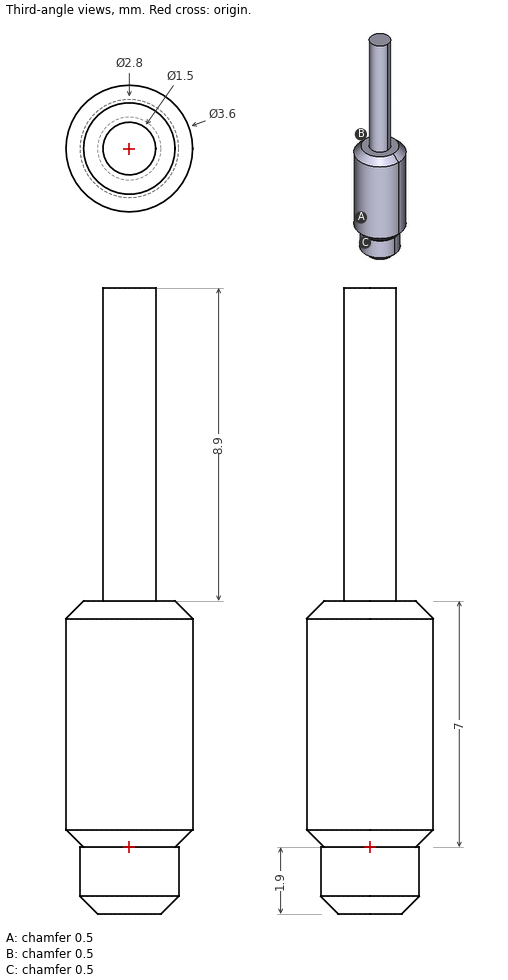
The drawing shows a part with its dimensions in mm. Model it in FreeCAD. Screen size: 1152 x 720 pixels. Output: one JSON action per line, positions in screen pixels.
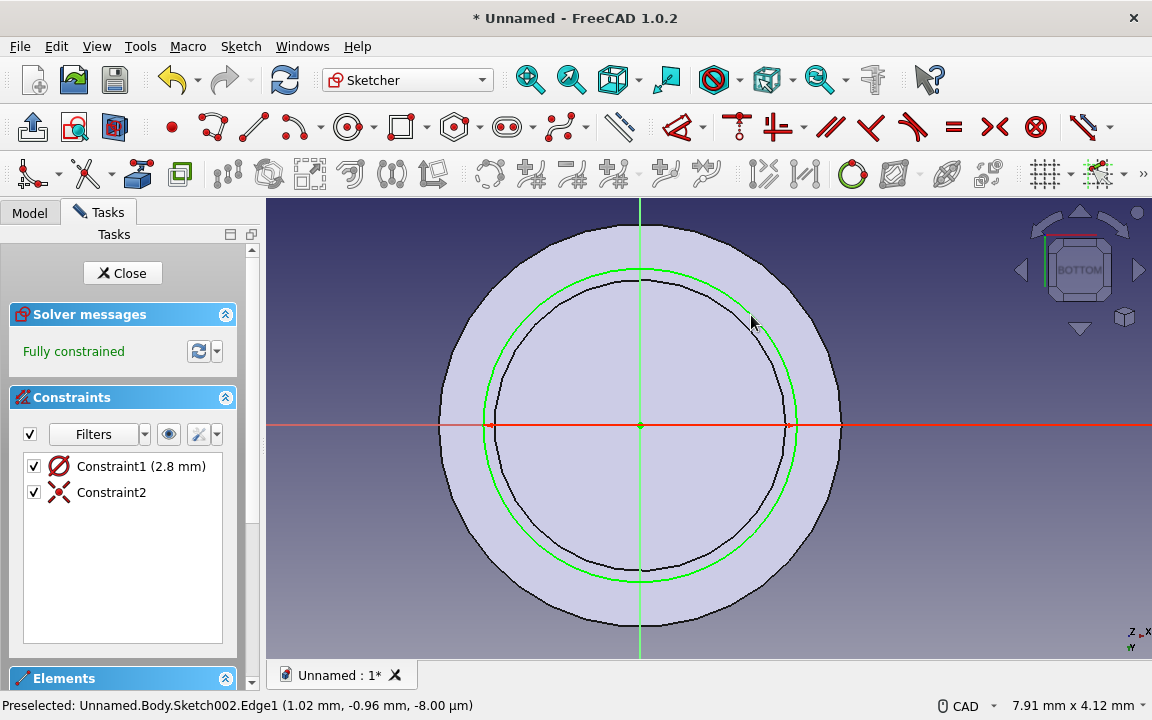
{"action": "left_click", "coordinate": [123, 273]}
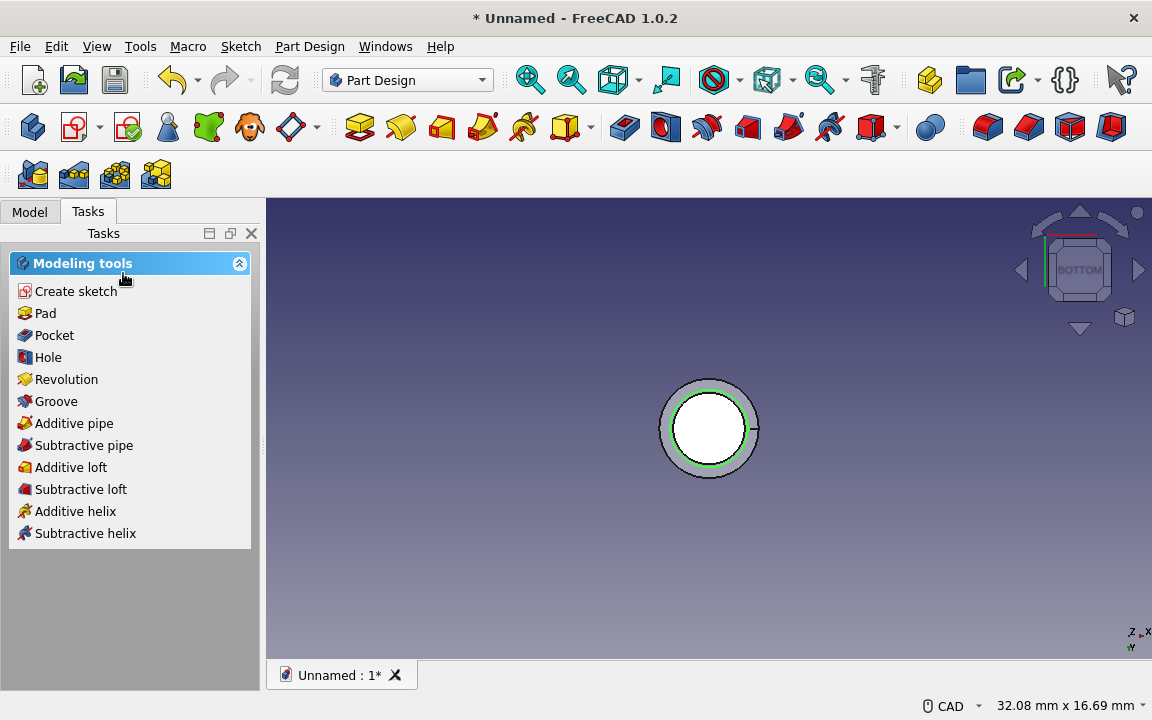
{"action": "left_click", "coordinate": [360, 128]}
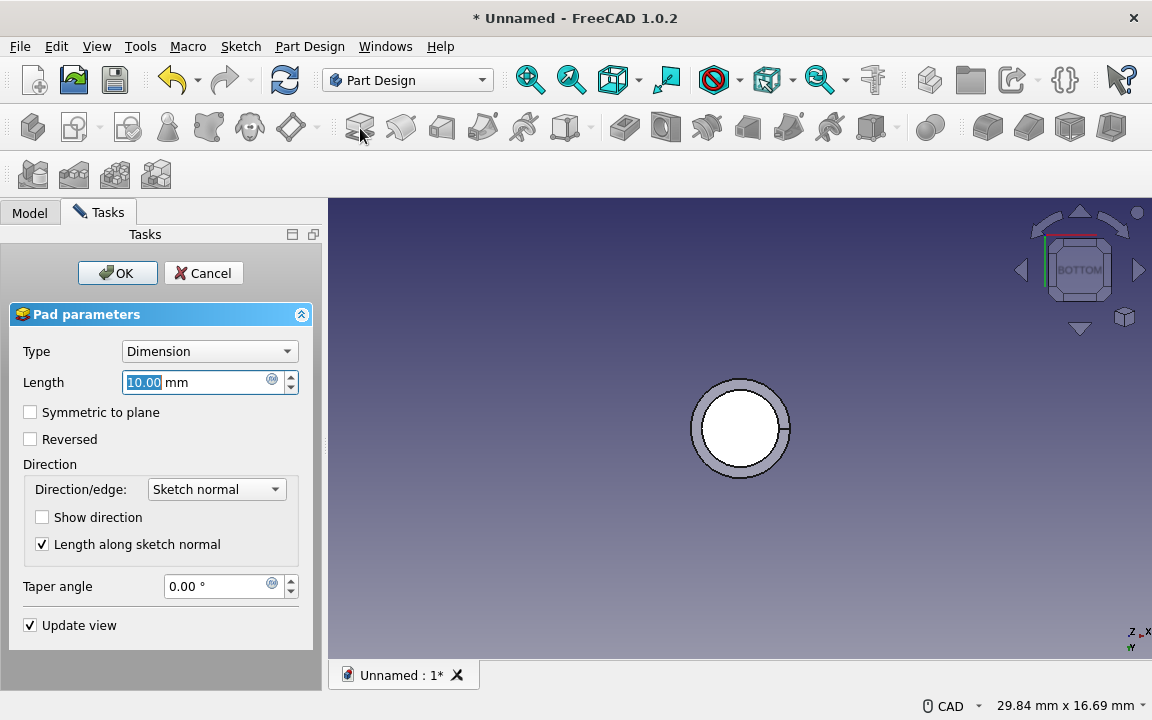
{"action": "type", "text": "1.9"}
{"action": "key", "text": "Tab"}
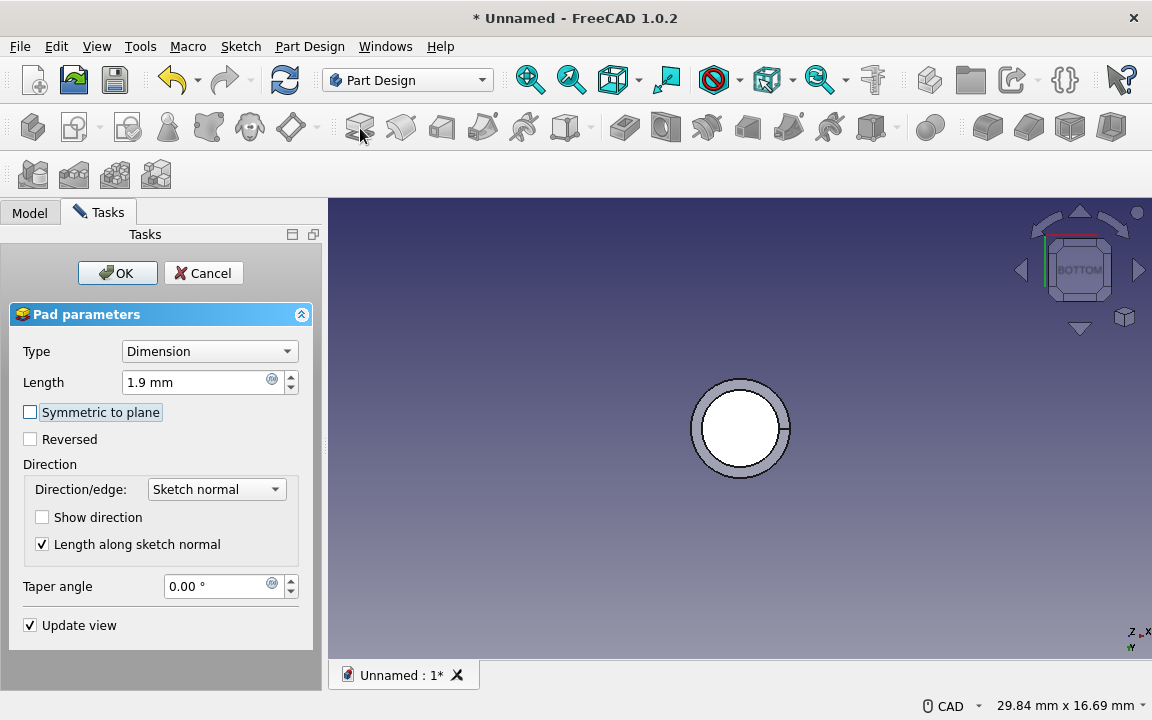
{"action": "left_click", "coordinate": [118, 273]}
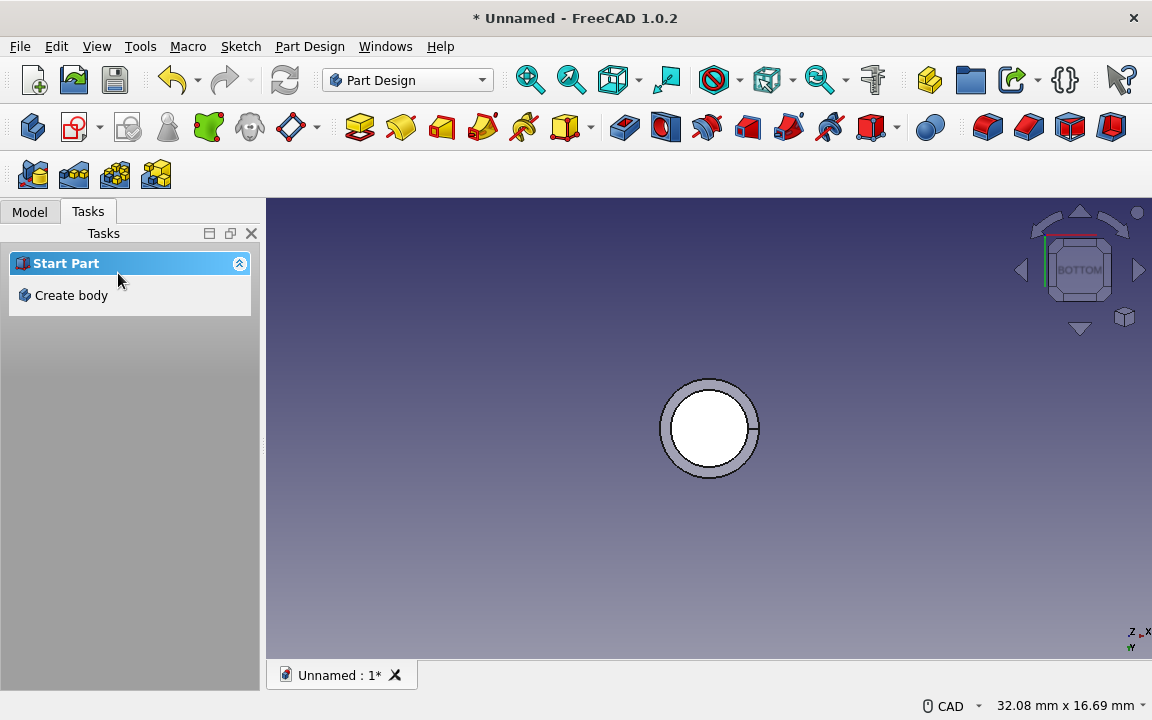
{"action": "key", "text": "v f"}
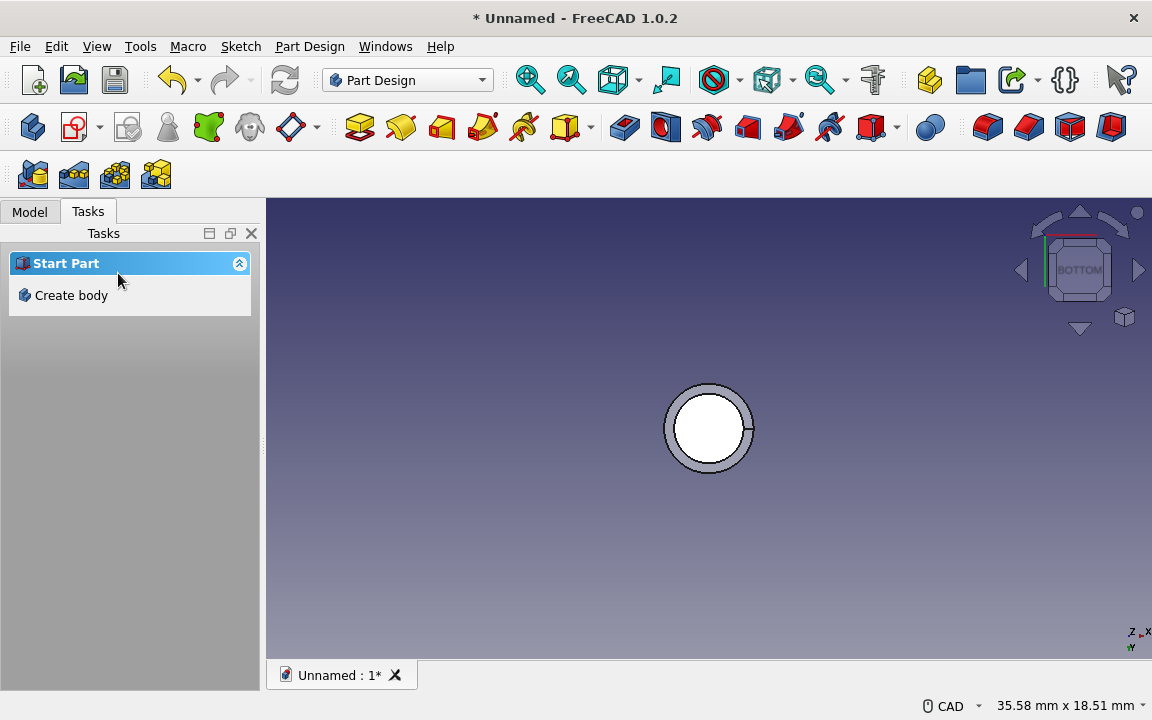
{"action": "left_click", "coordinate": [674, 427]}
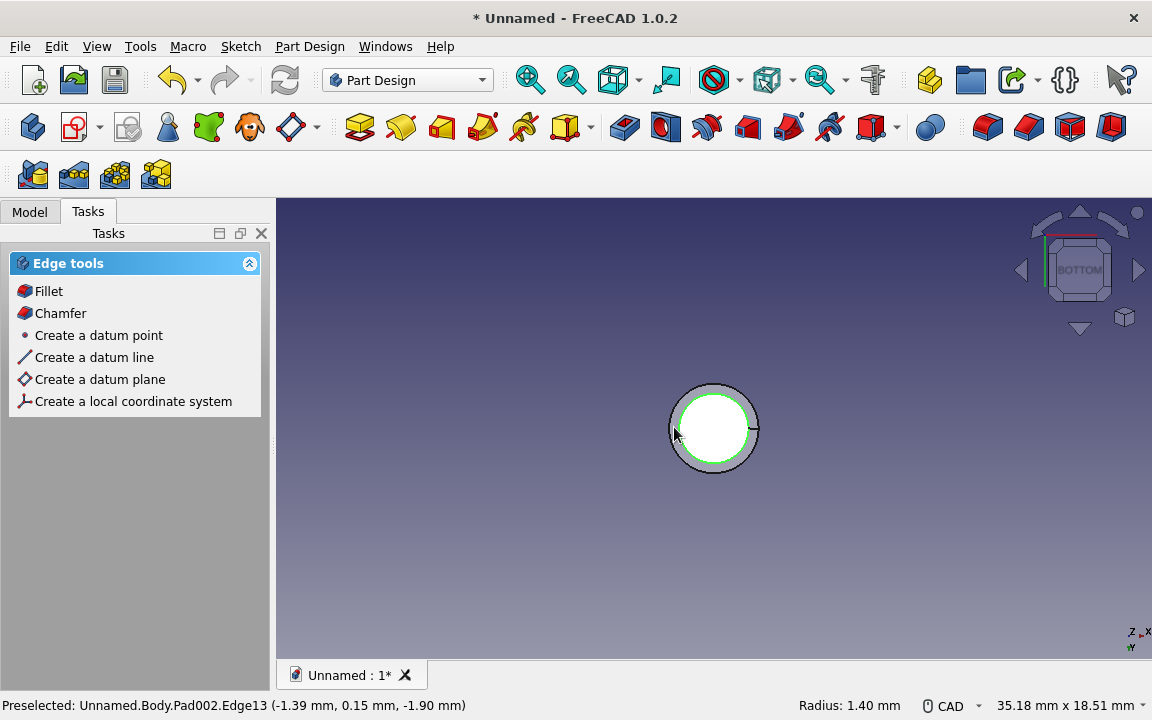
{"action": "left_click", "coordinate": [1029, 128]}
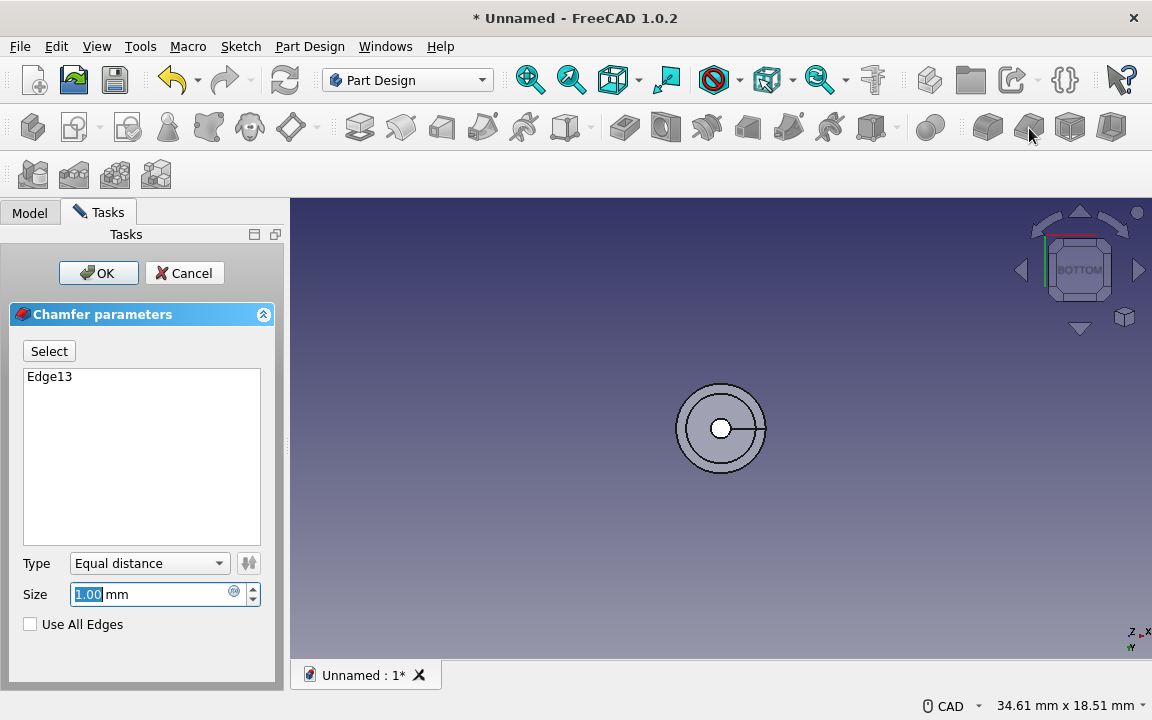
{"action": "type", "text": "0.5"}
{"action": "key", "text": "Tab"}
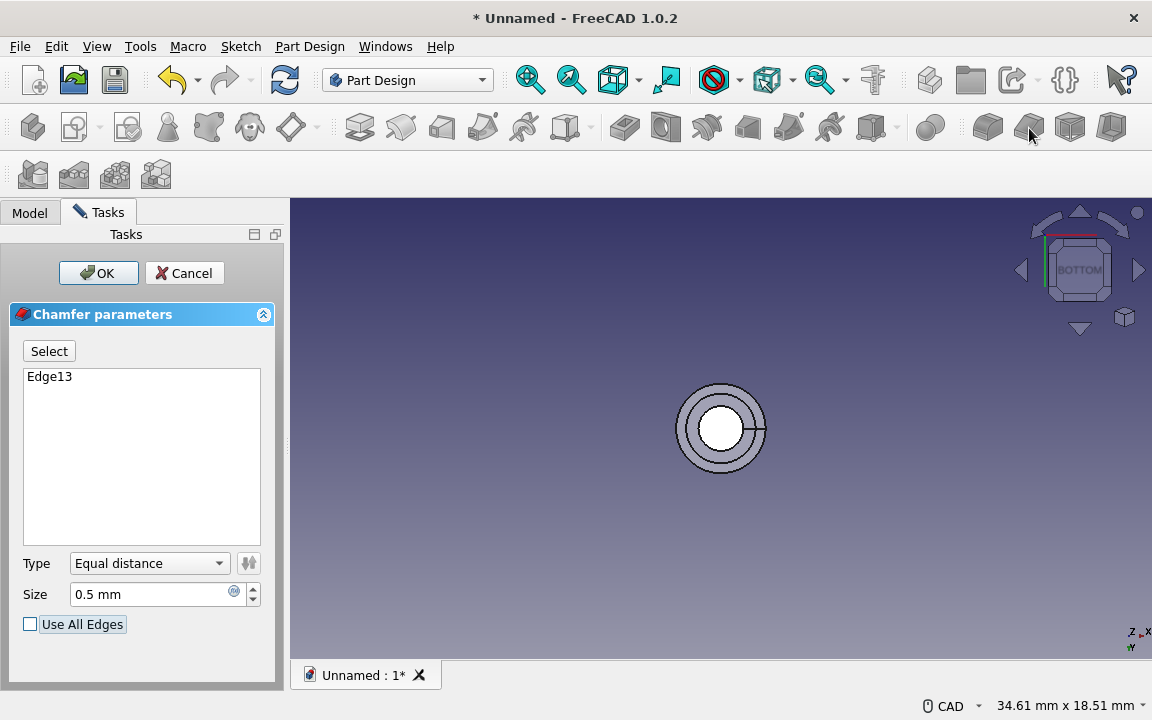
{"action": "left_click", "coordinate": [99, 273]}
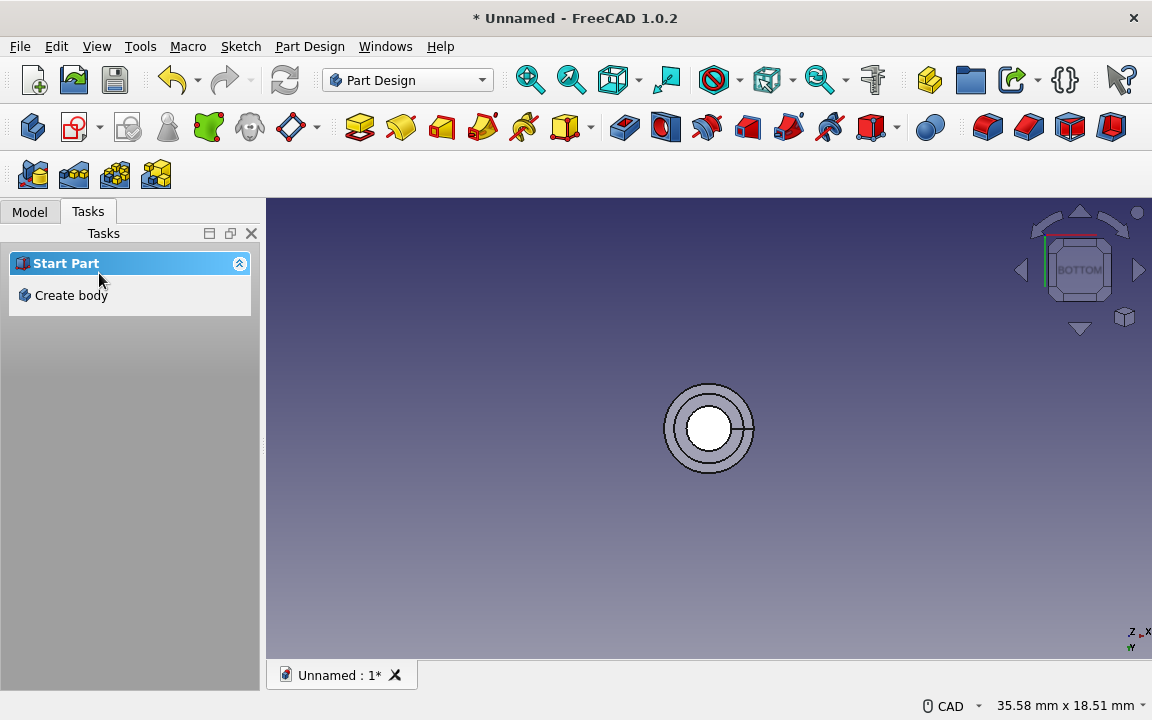
{"action": "key", "text": "0"}